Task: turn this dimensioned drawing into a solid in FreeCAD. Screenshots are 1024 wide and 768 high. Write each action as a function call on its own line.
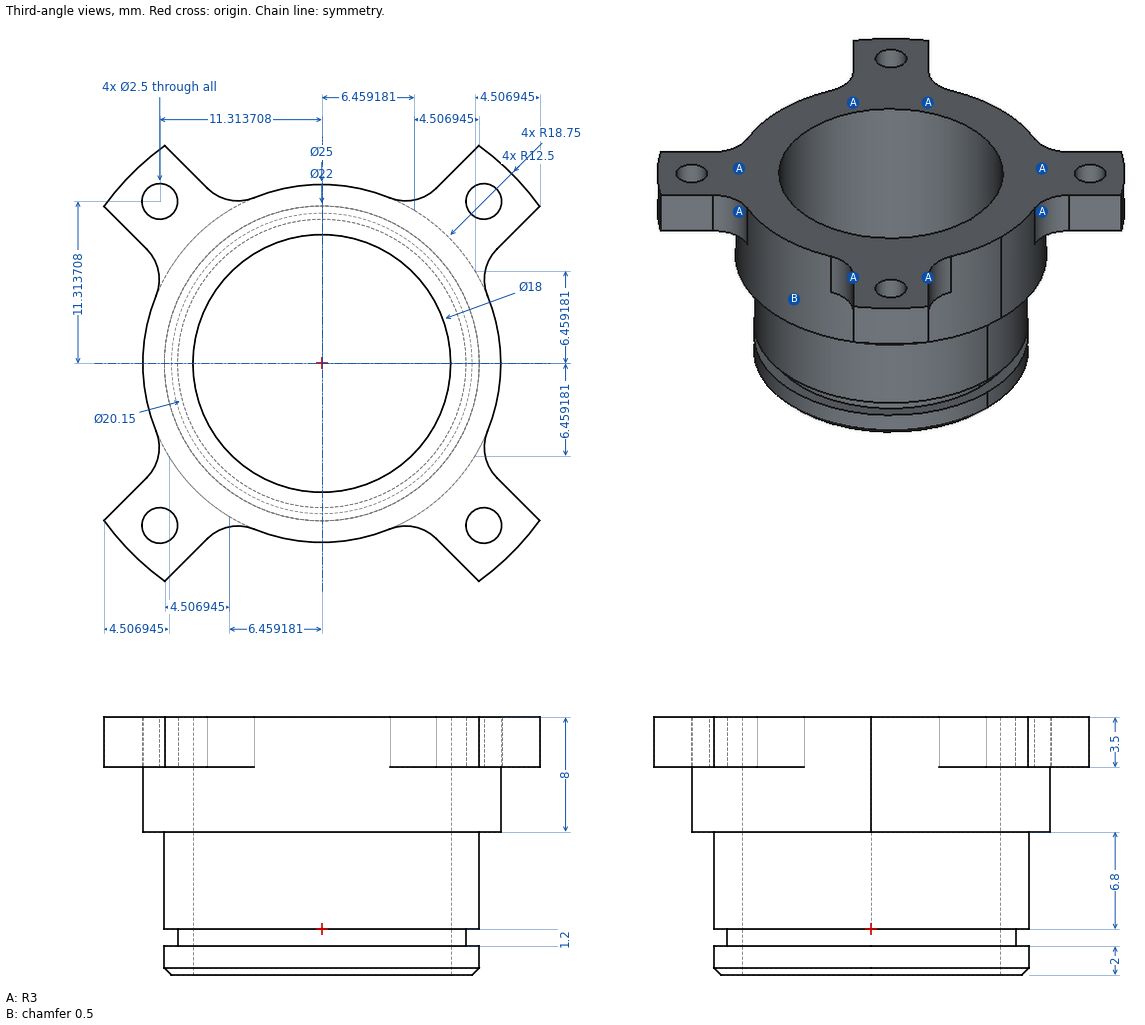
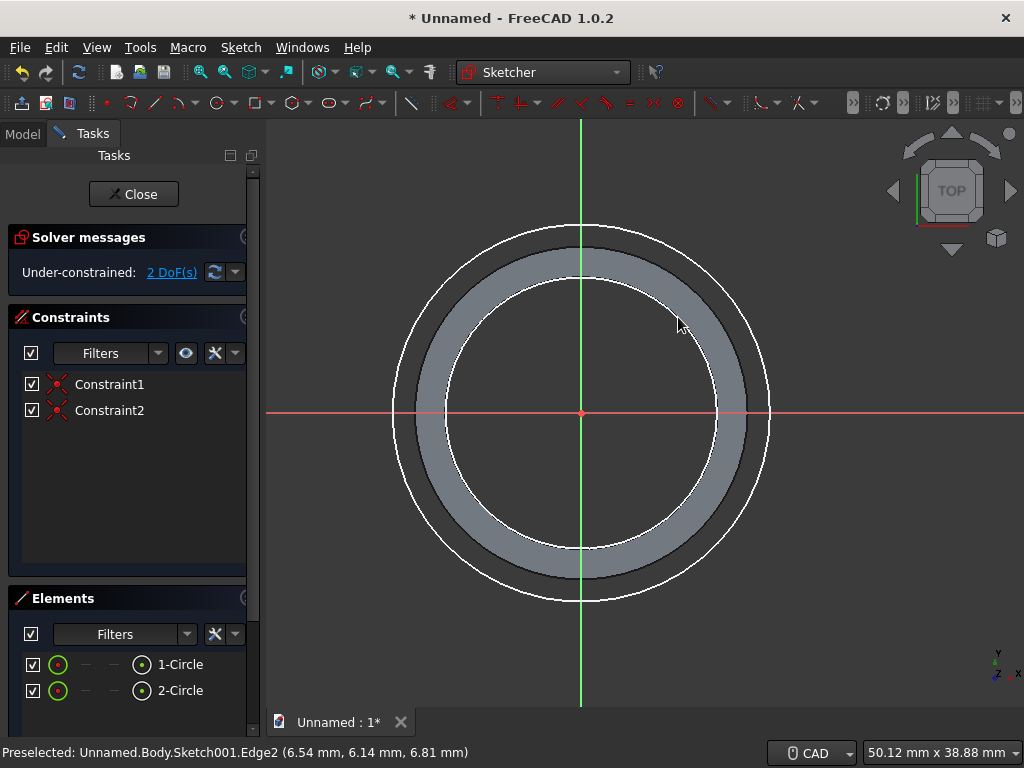
click(450, 104)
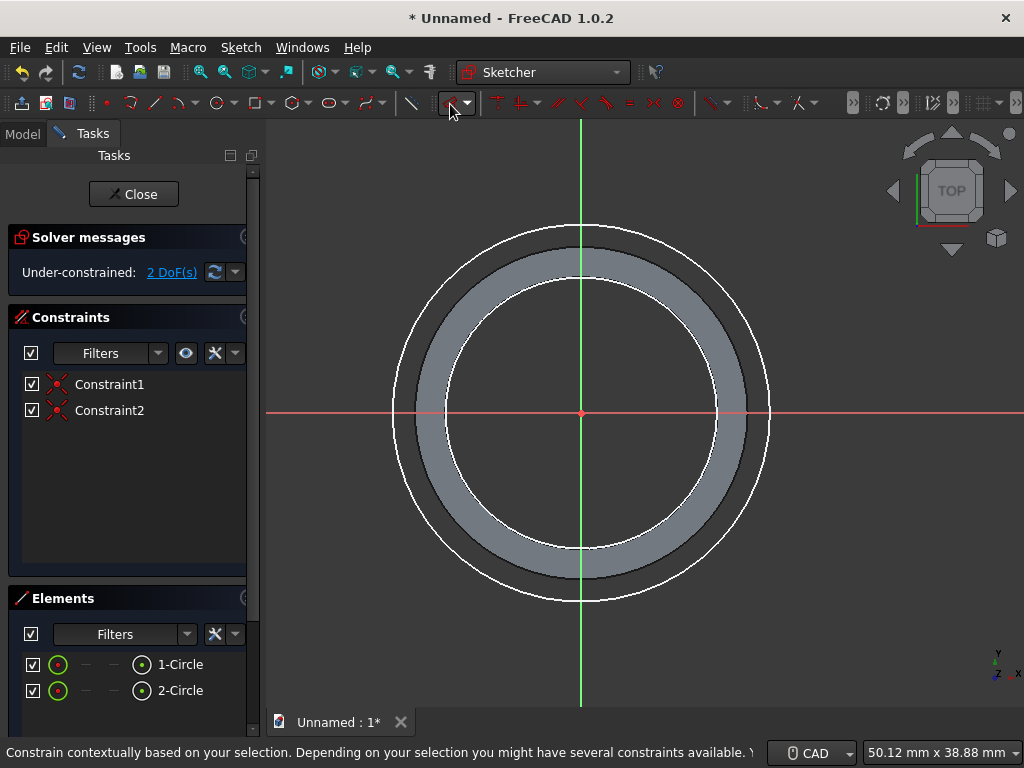
click(714, 279)
click(737, 256)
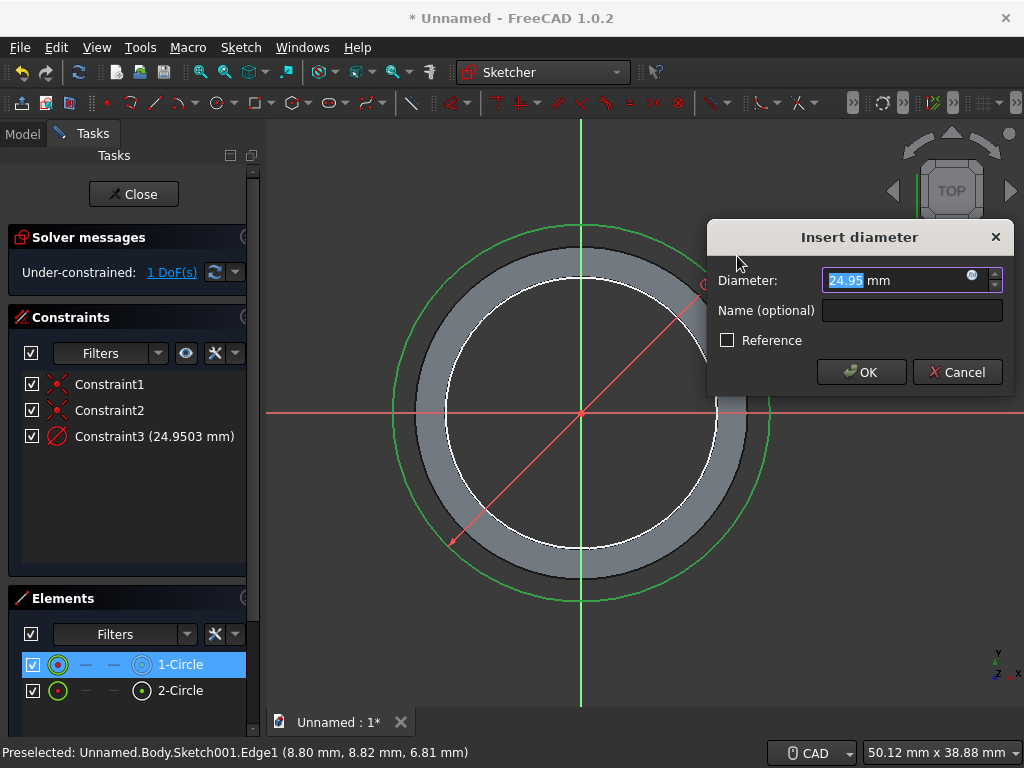
text(25)
key(Return)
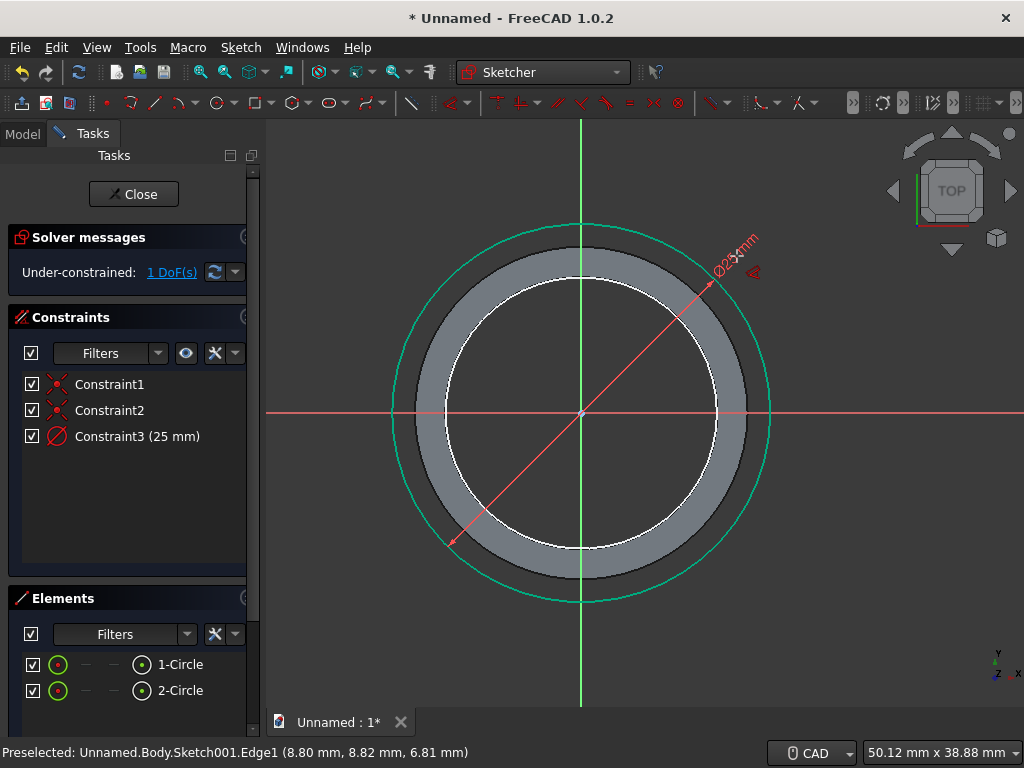
click(677, 317)
click(700, 294)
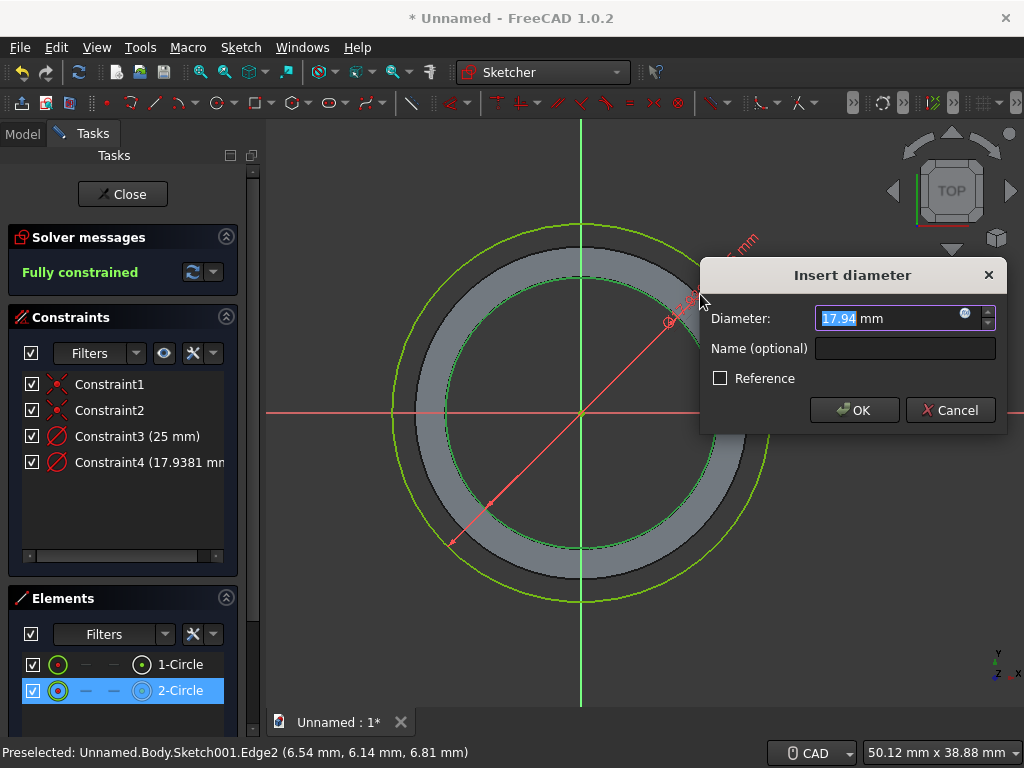
text(18)
key(Return)
key(Escape)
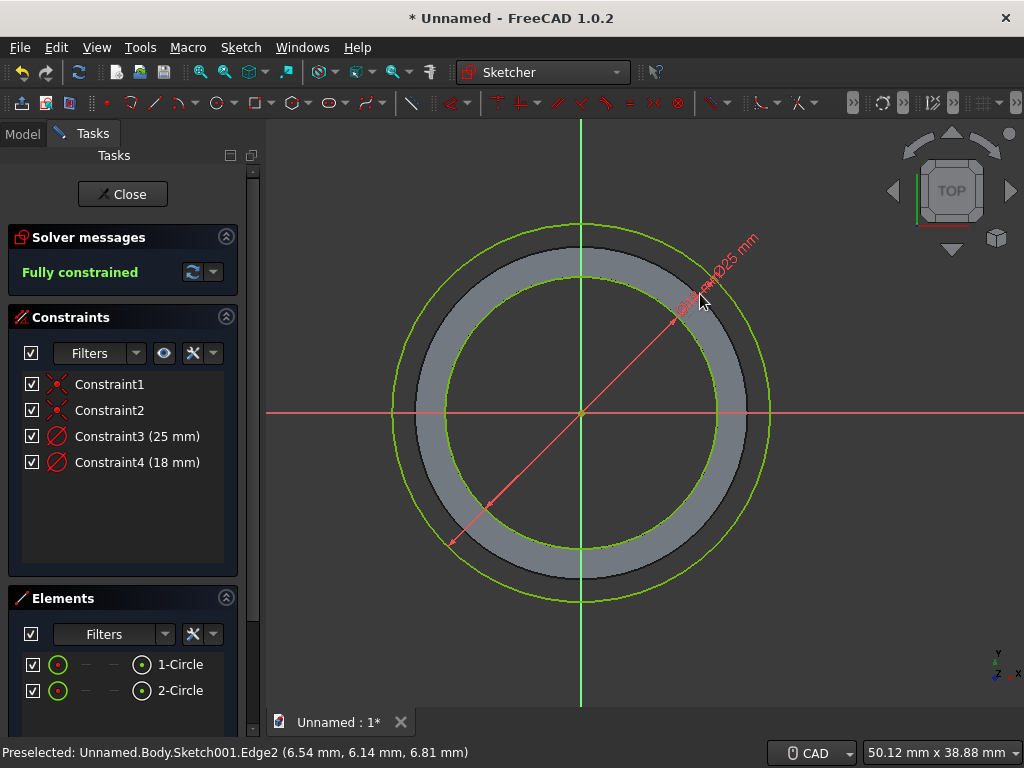
click(123, 194)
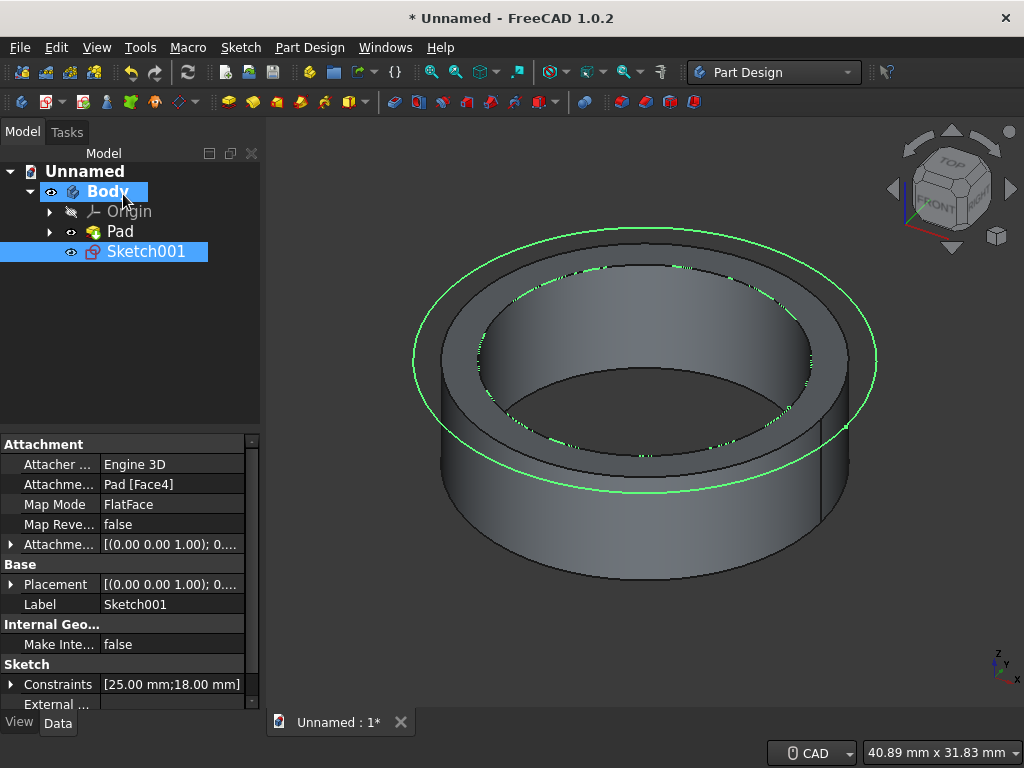
click(230, 102)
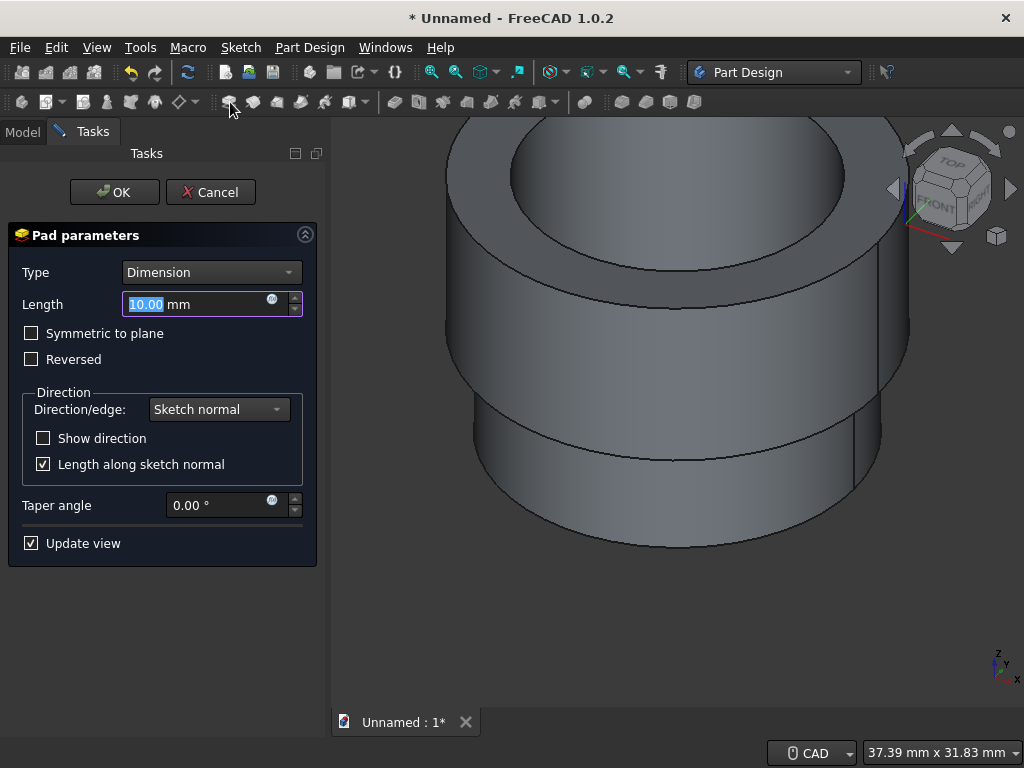
text(8)
key(Tab)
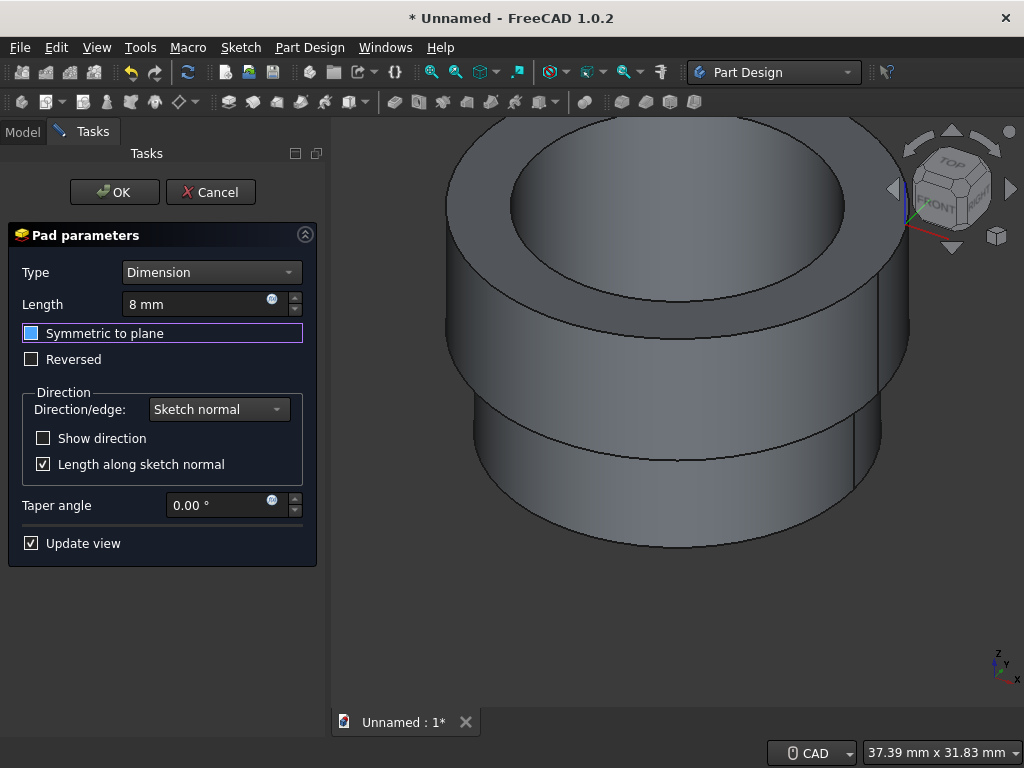
click(115, 192)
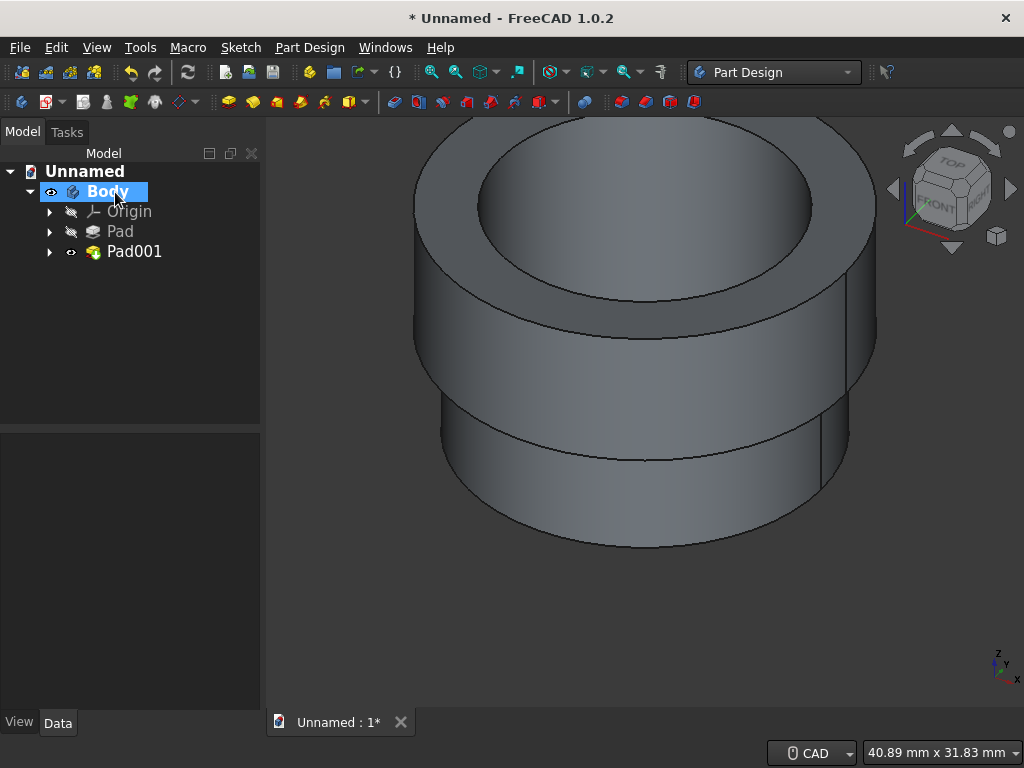
click(432, 72)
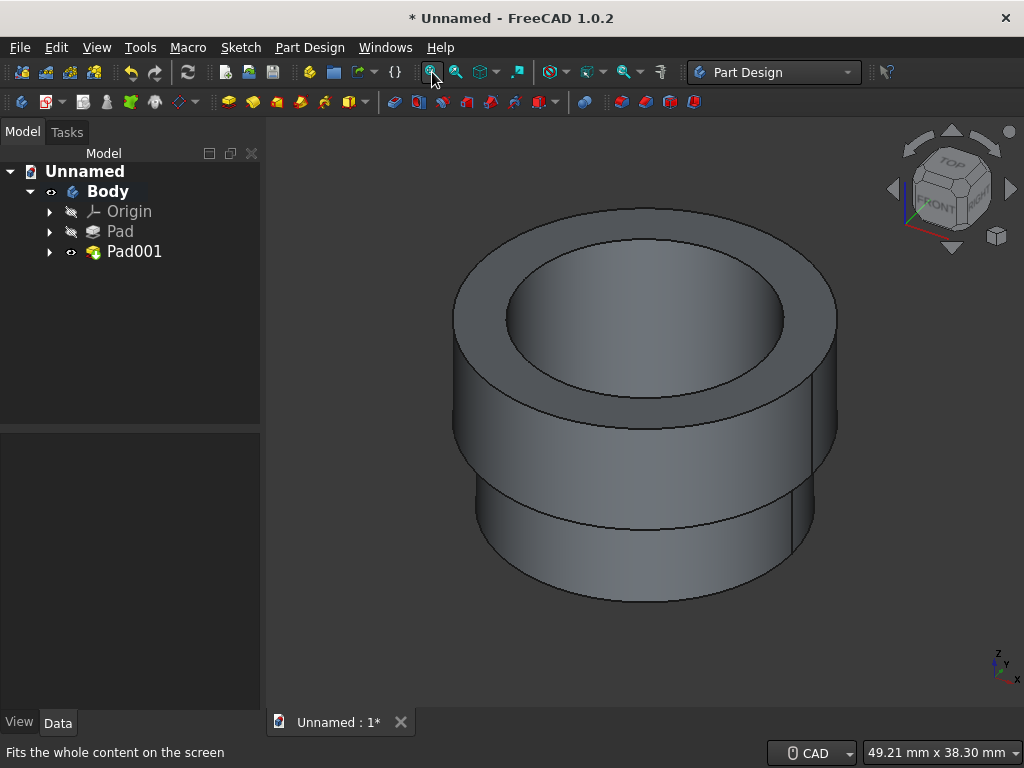
click(788, 365)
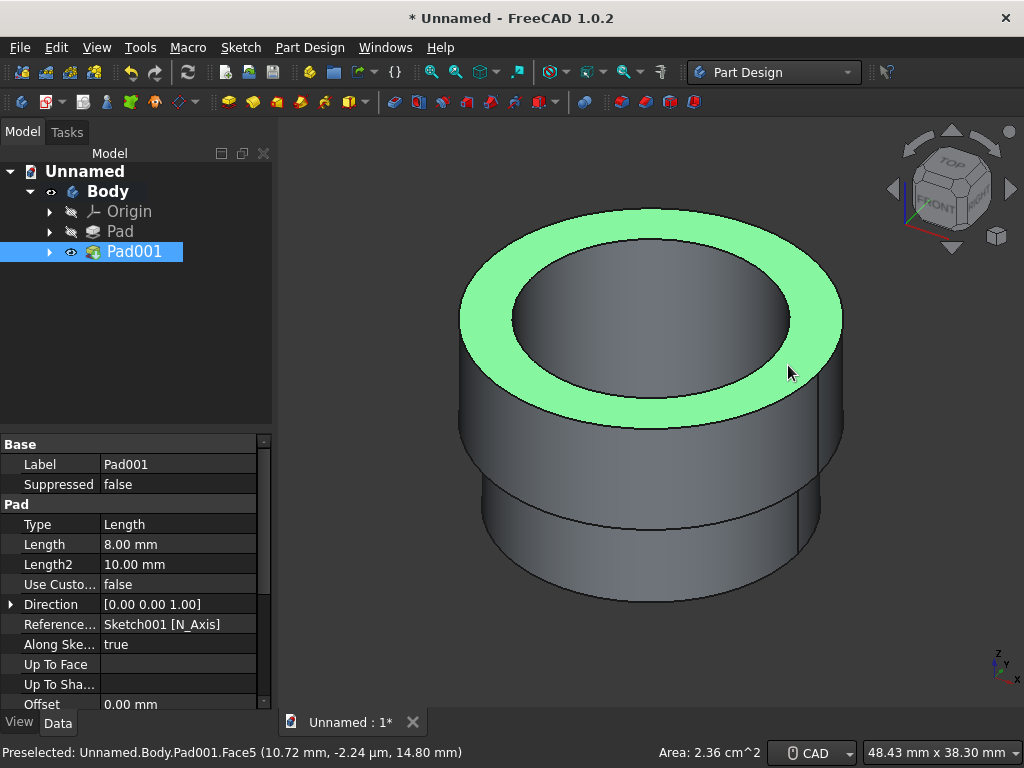
click(46, 102)